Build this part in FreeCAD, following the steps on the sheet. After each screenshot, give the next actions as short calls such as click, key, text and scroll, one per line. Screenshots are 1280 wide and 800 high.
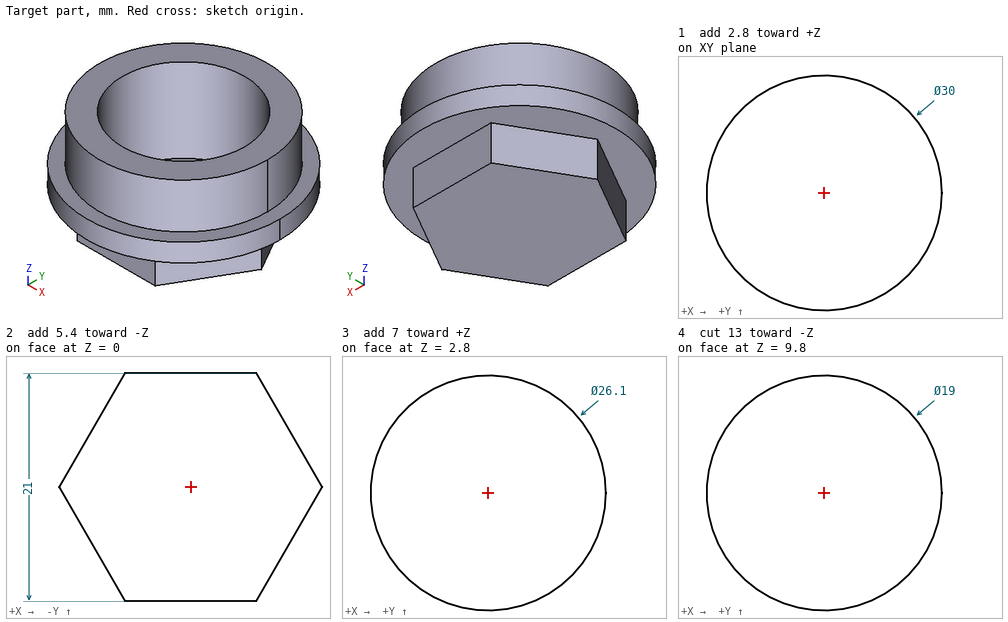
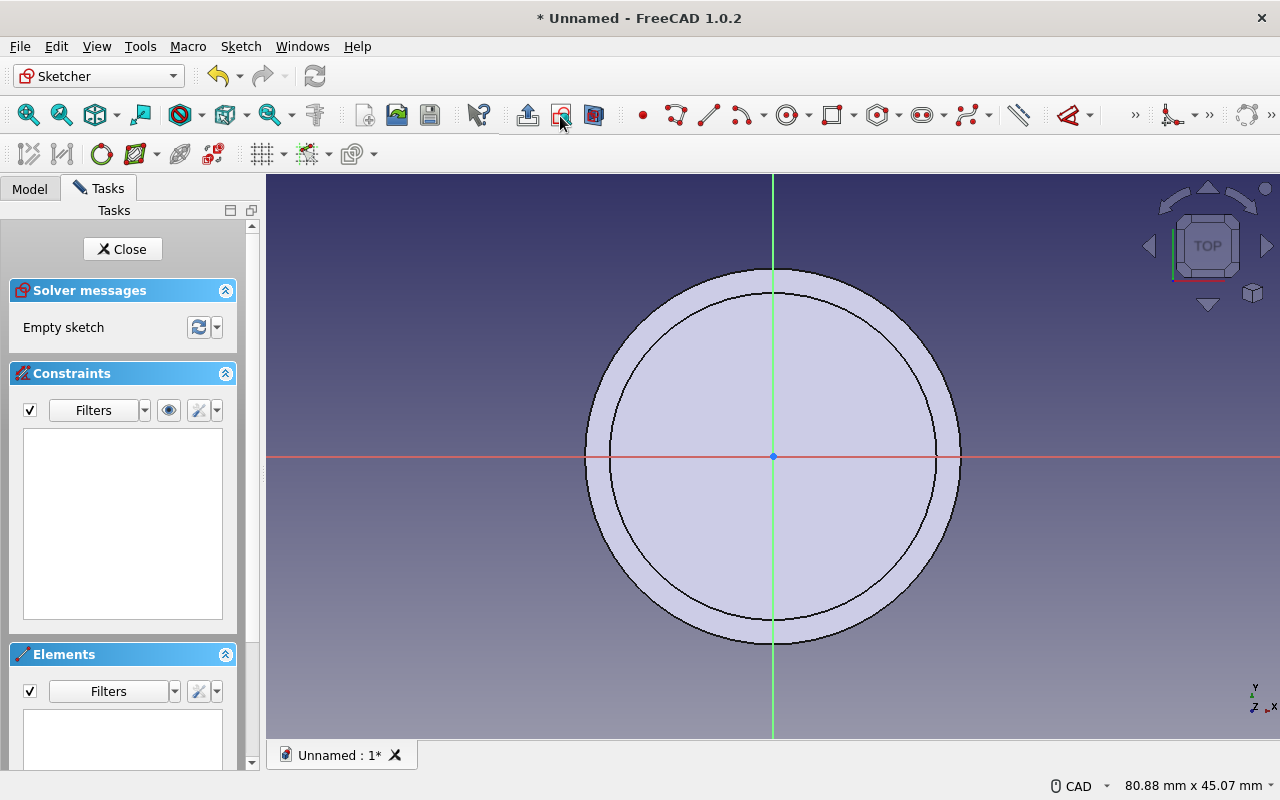
scroll(912, 456, up, 2)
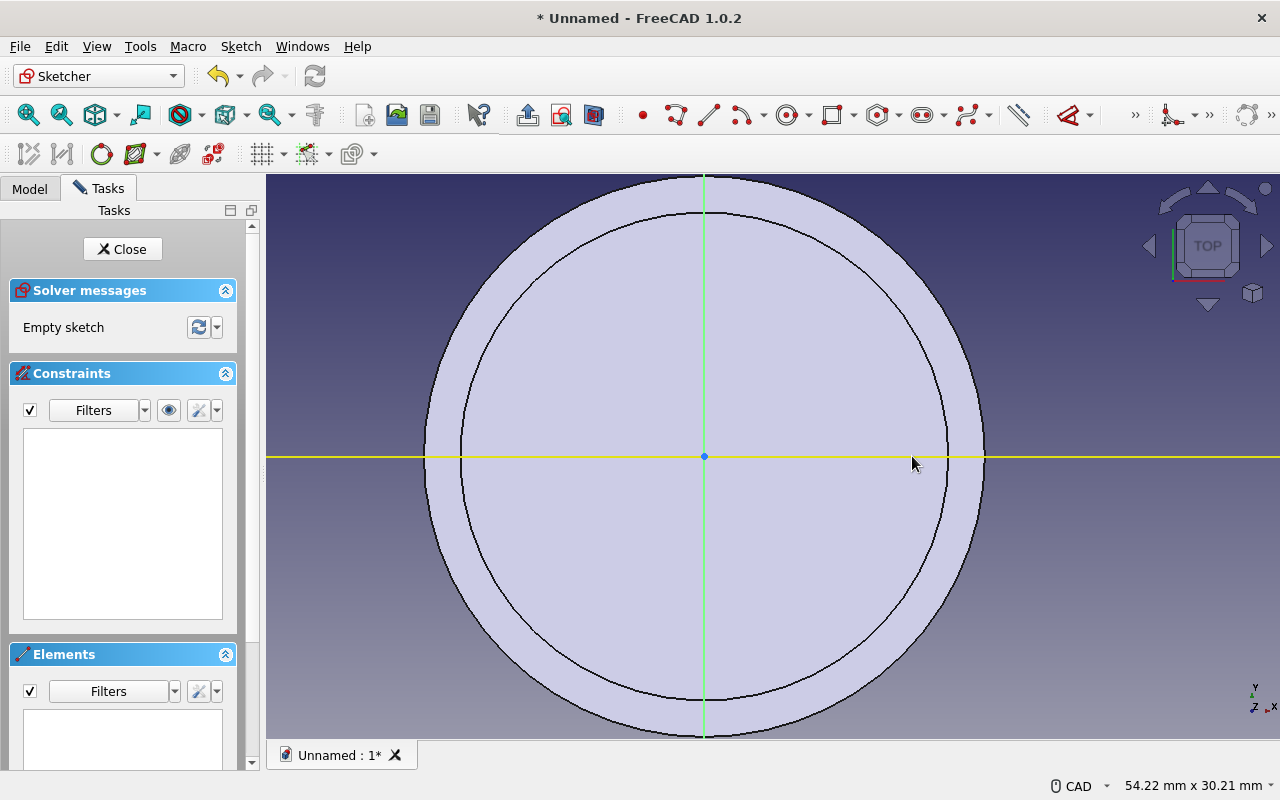
click(786, 116)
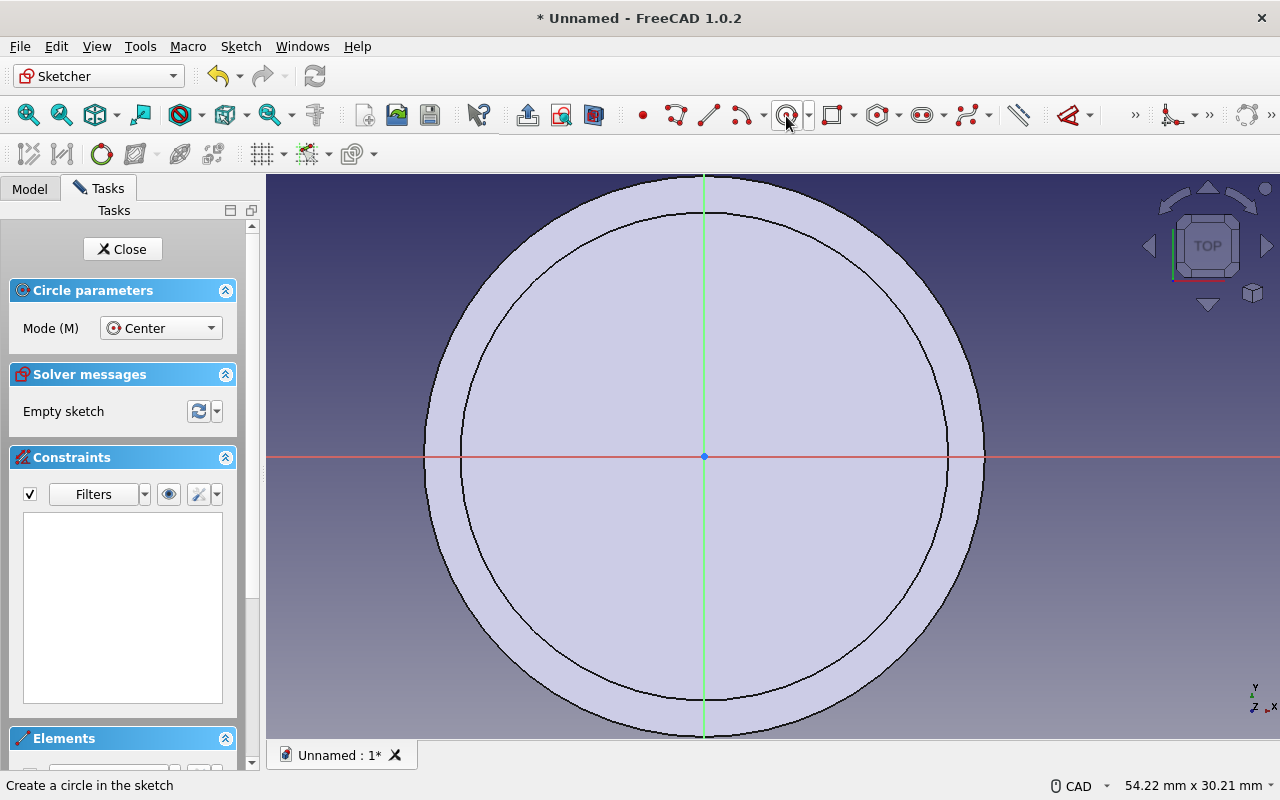
click(704, 456)
move(830, 331)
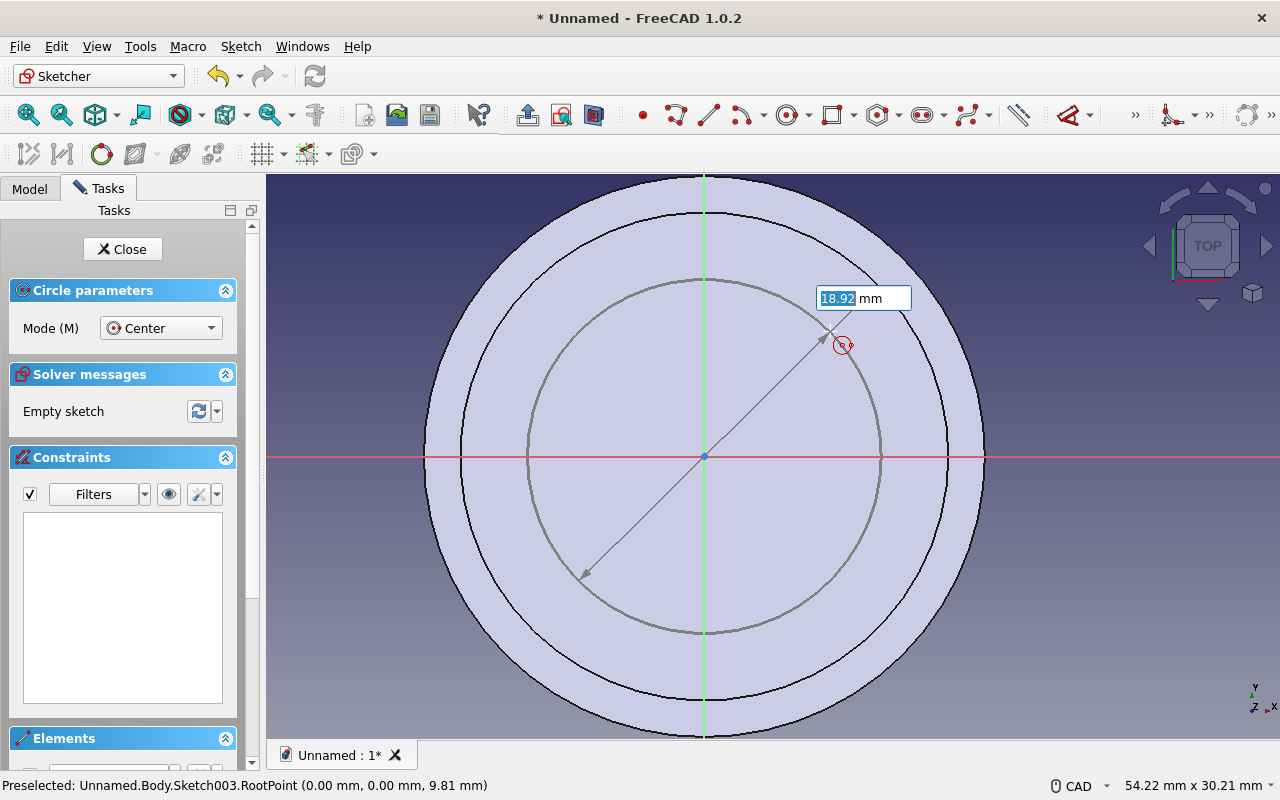
text(19)
key(Return)
key(Escape)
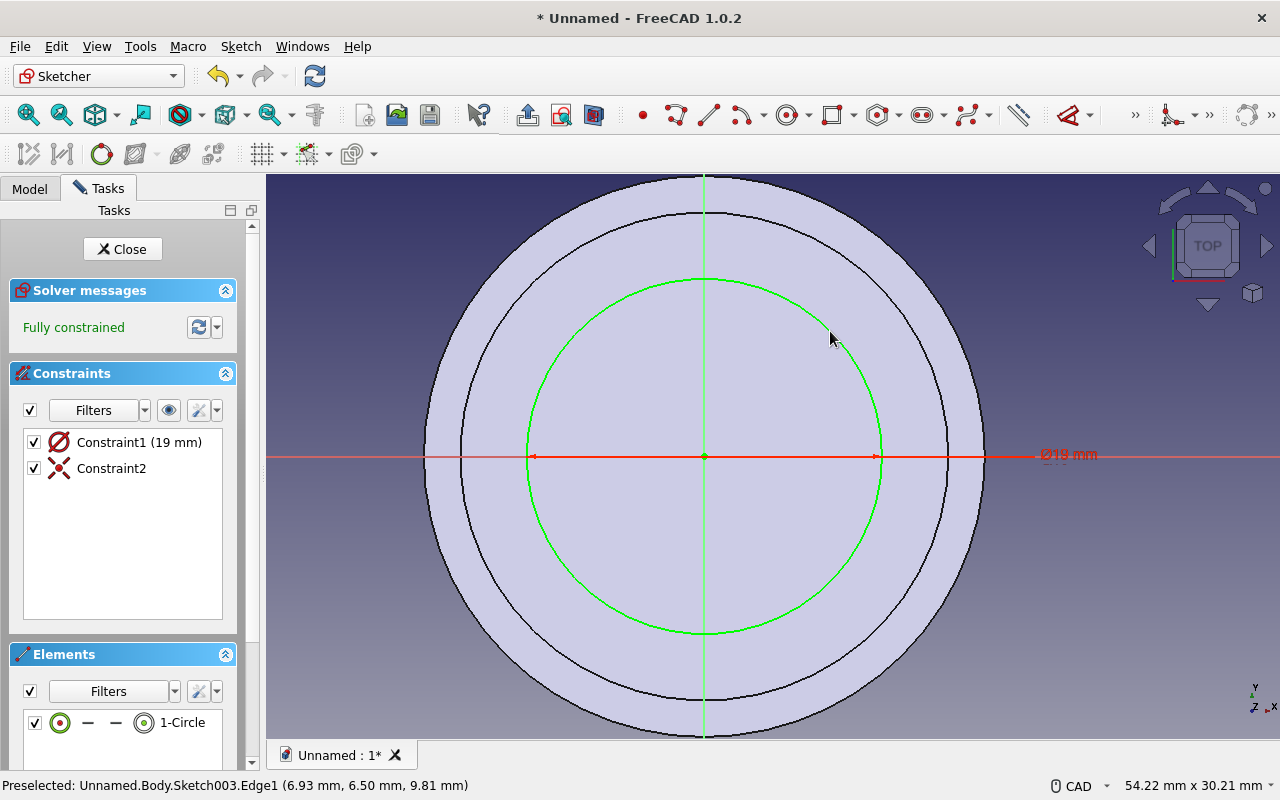
click(123, 249)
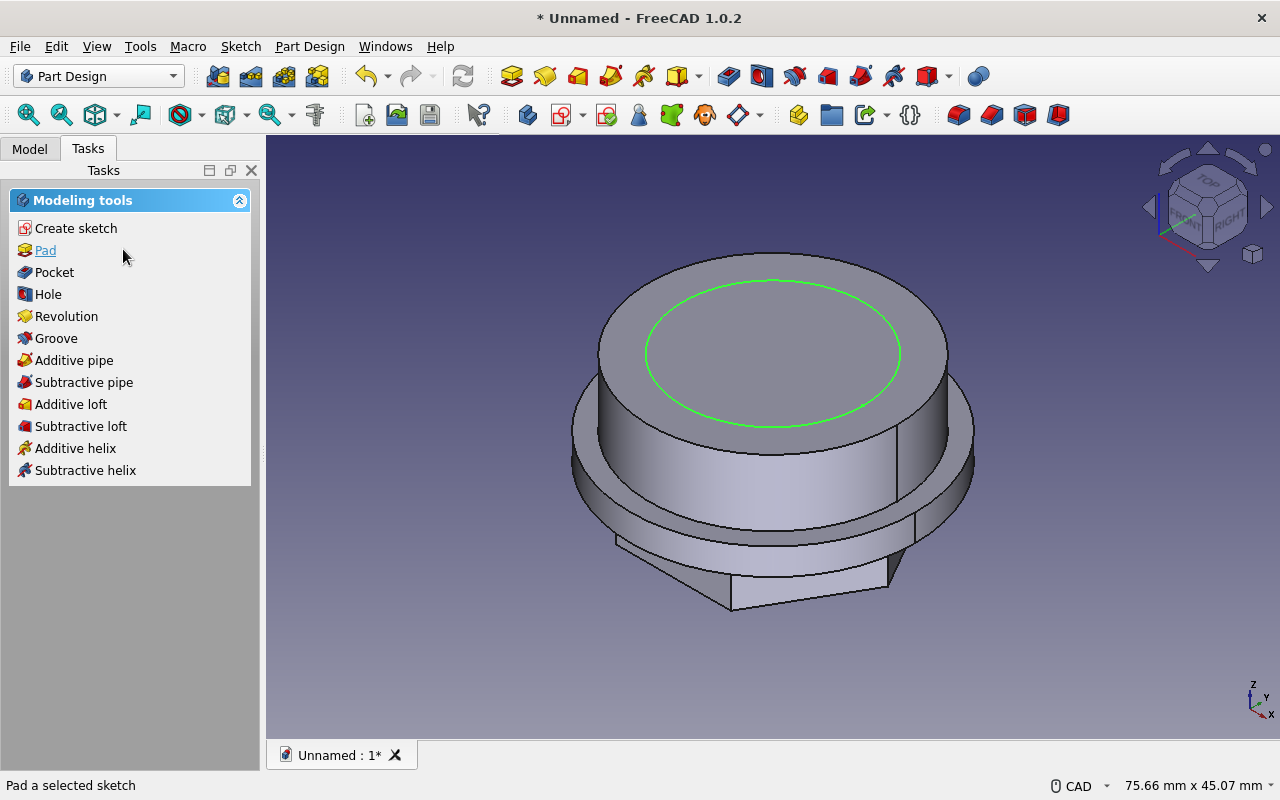
click(729, 76)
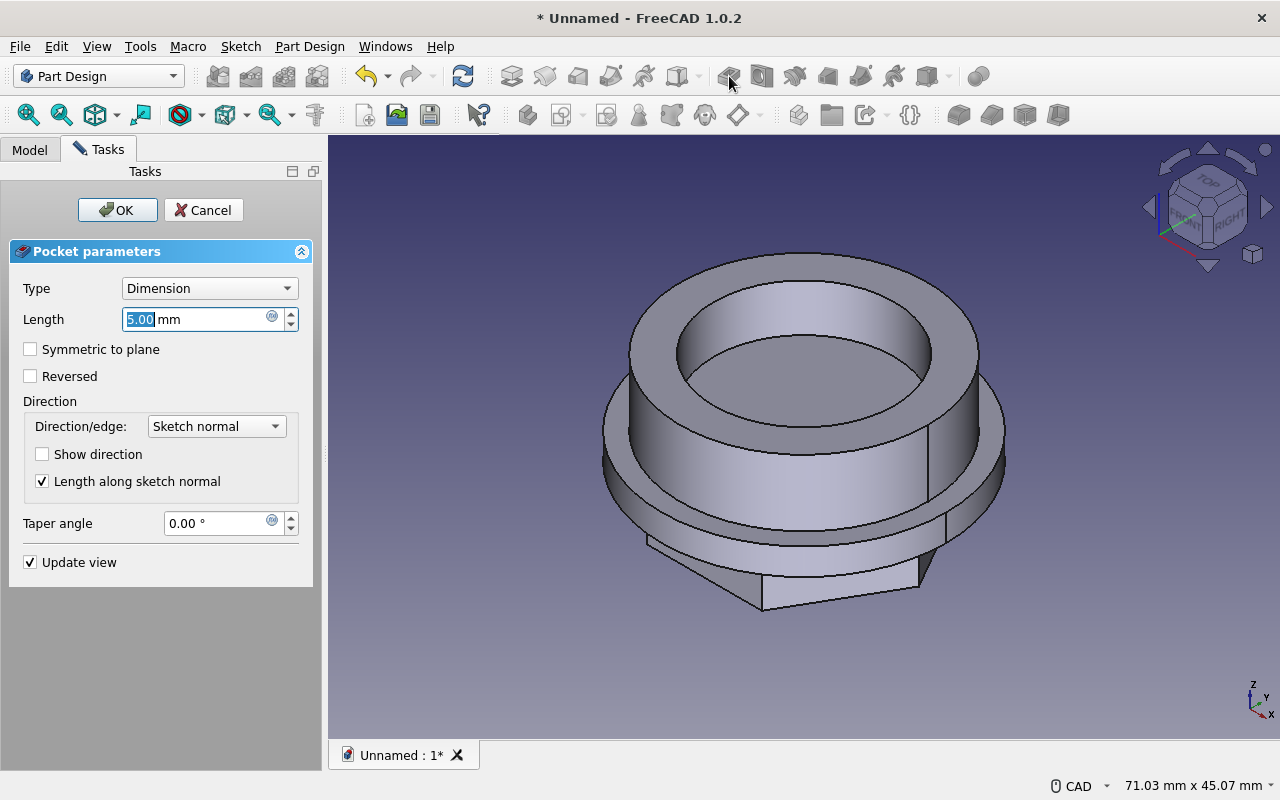
text(13)
key(Tab)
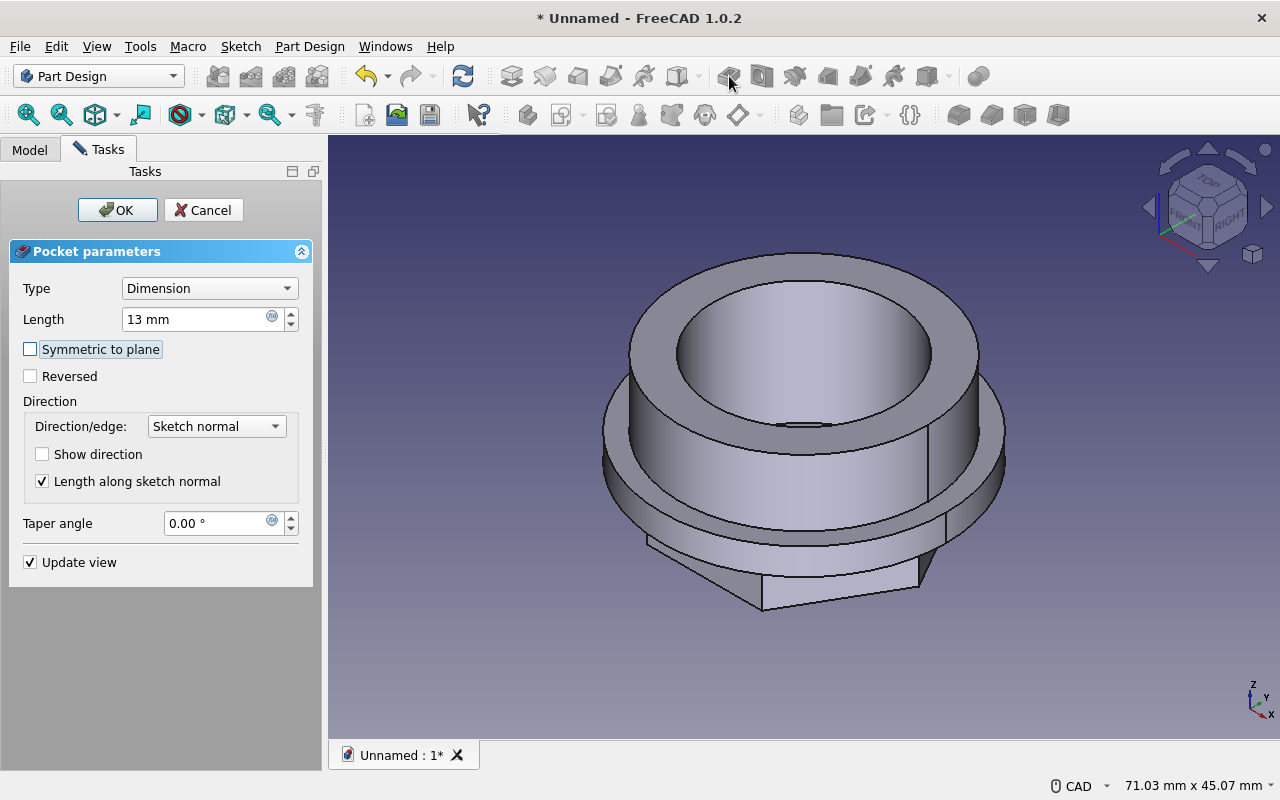
click(118, 210)